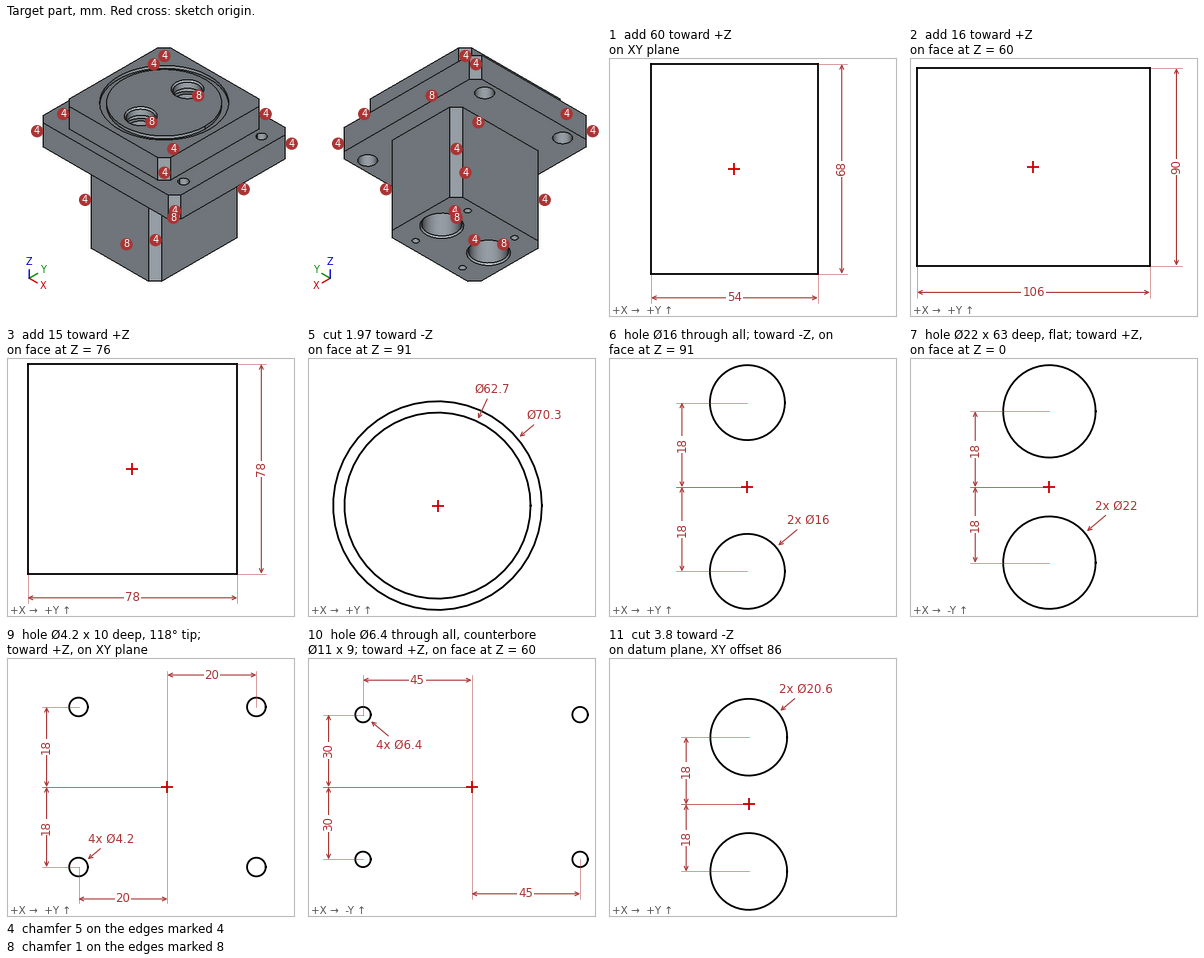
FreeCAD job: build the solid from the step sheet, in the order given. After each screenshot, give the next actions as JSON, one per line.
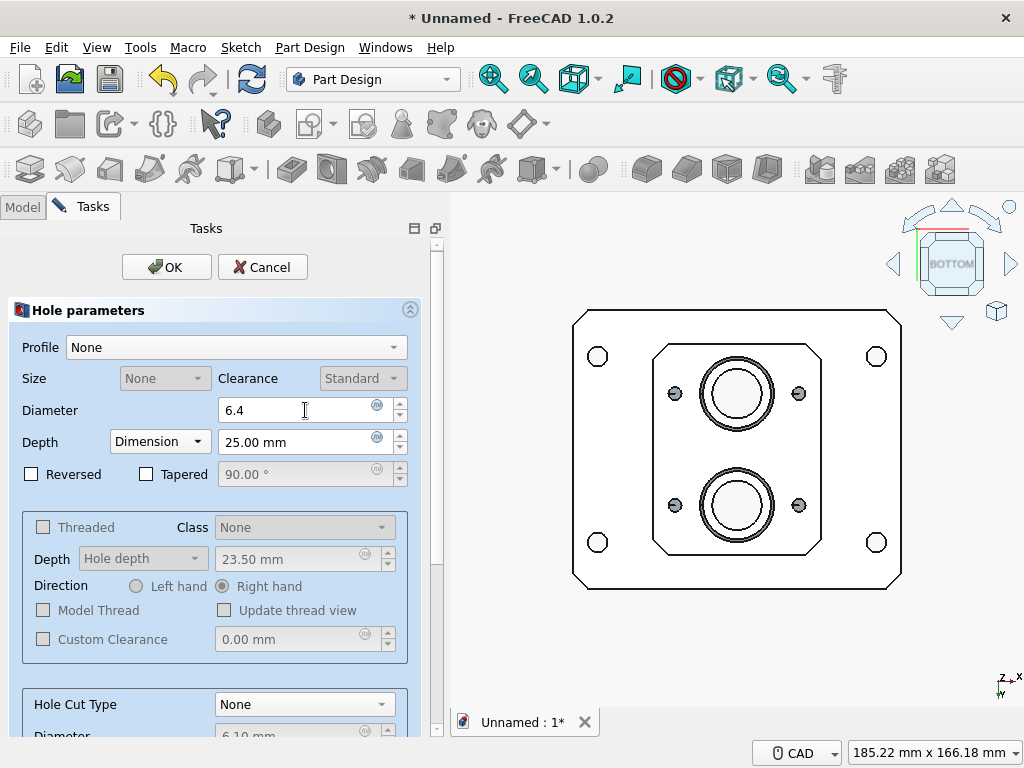
{"action": "left_click", "coordinate": [161, 442]}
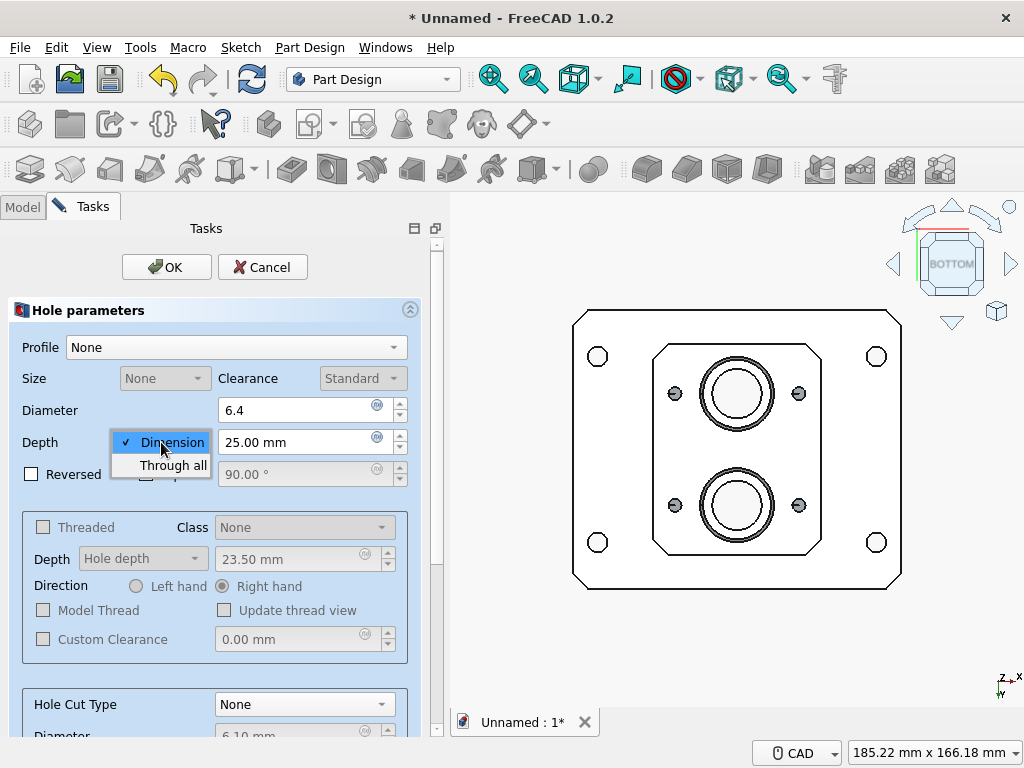
{"action": "left_click", "coordinate": [160, 466]}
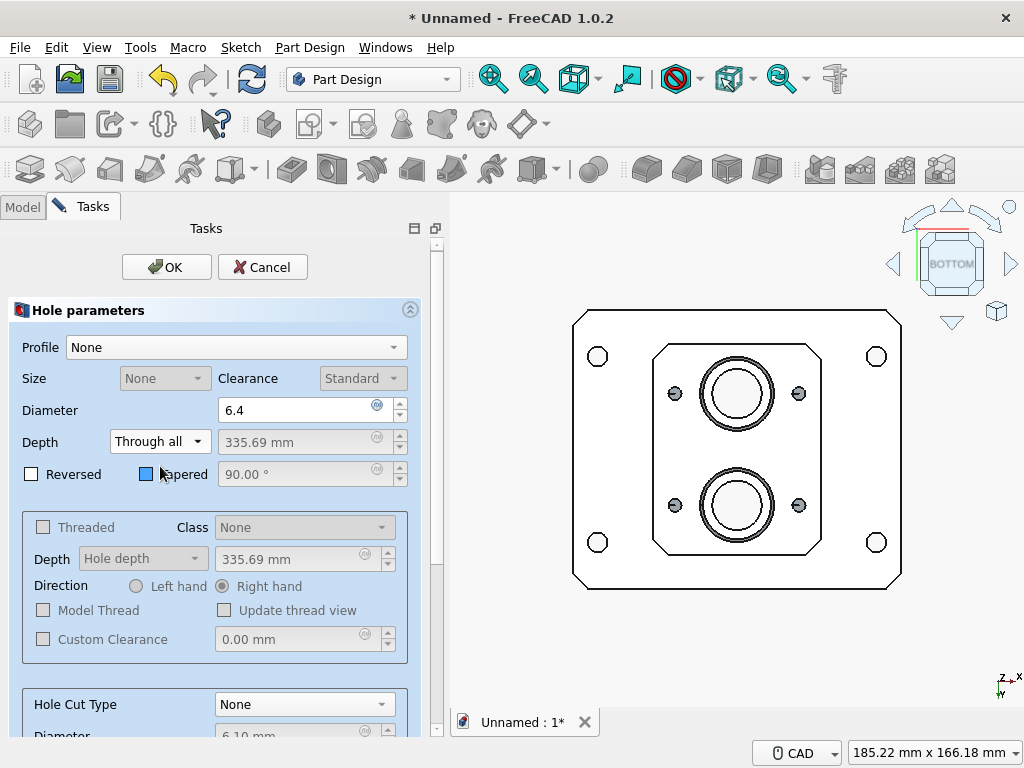
{"action": "left_click", "coordinate": [306, 704]}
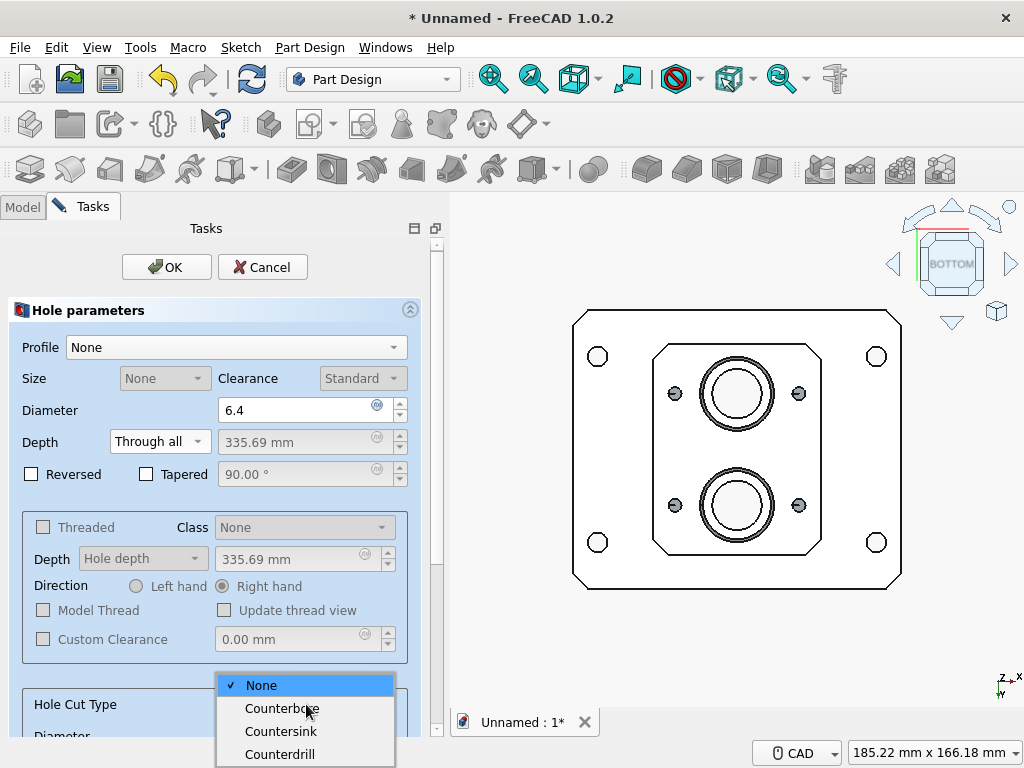
{"action": "left_click", "coordinate": [304, 708]}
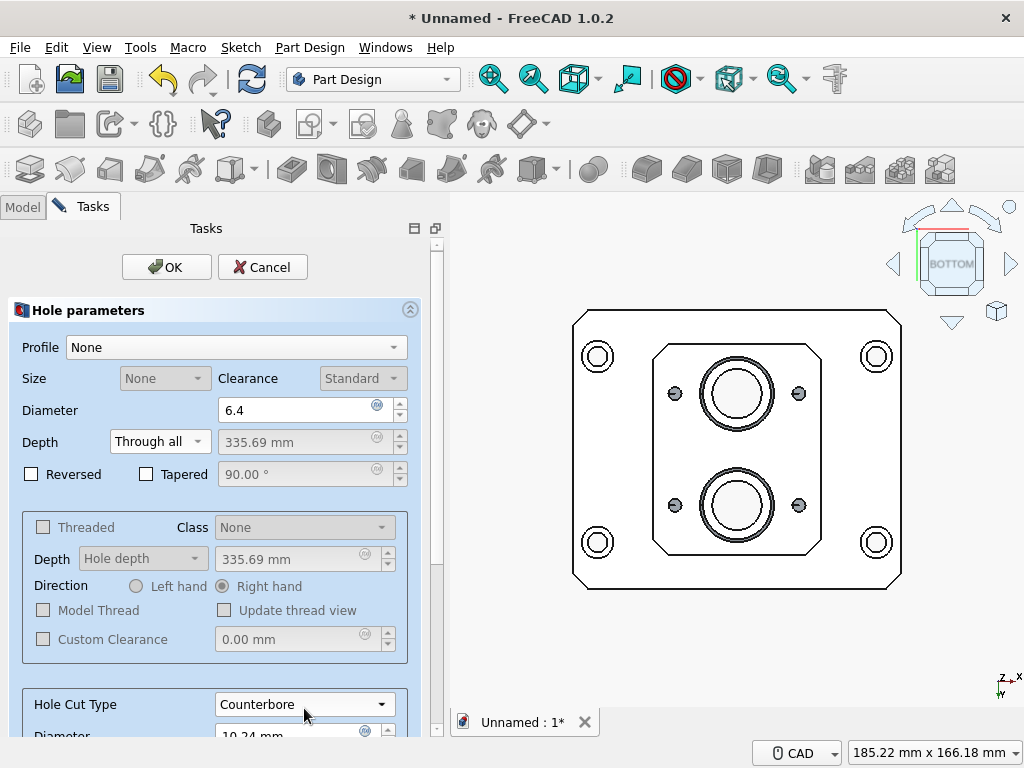
{"action": "scroll", "coordinate": [437, 487], "scroll_direction": "down", "scroll_amount": 2}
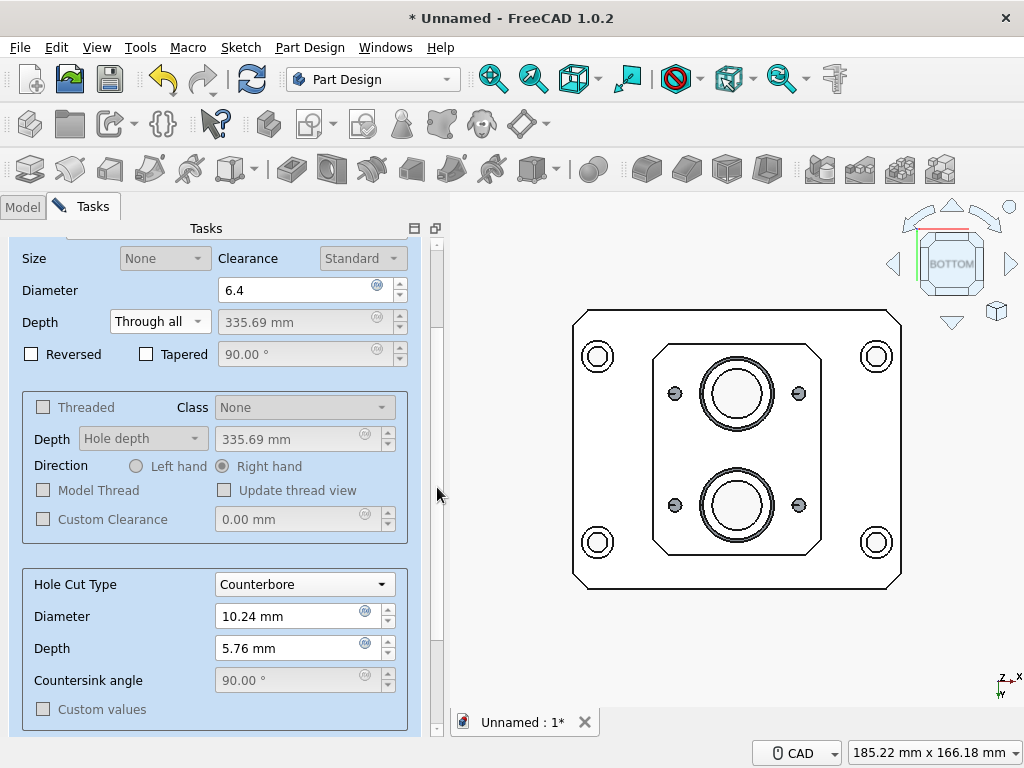
{"action": "triple_click", "coordinate": [298, 616]}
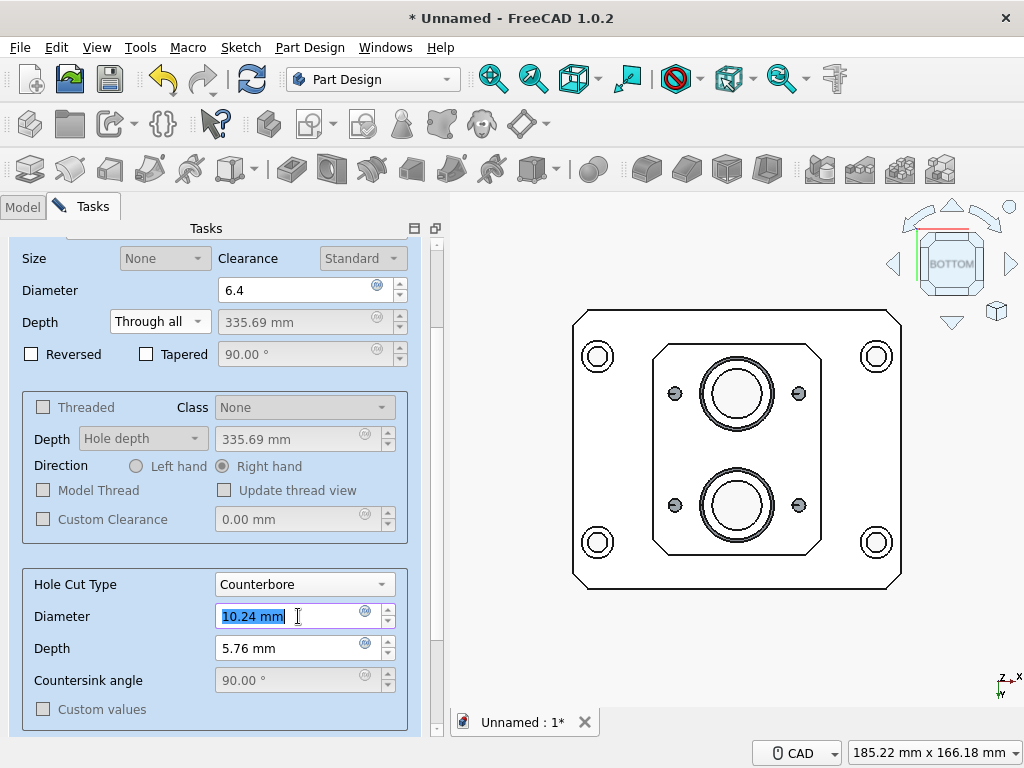
{"action": "type", "text": "11"}
{"action": "key", "text": "Tab"}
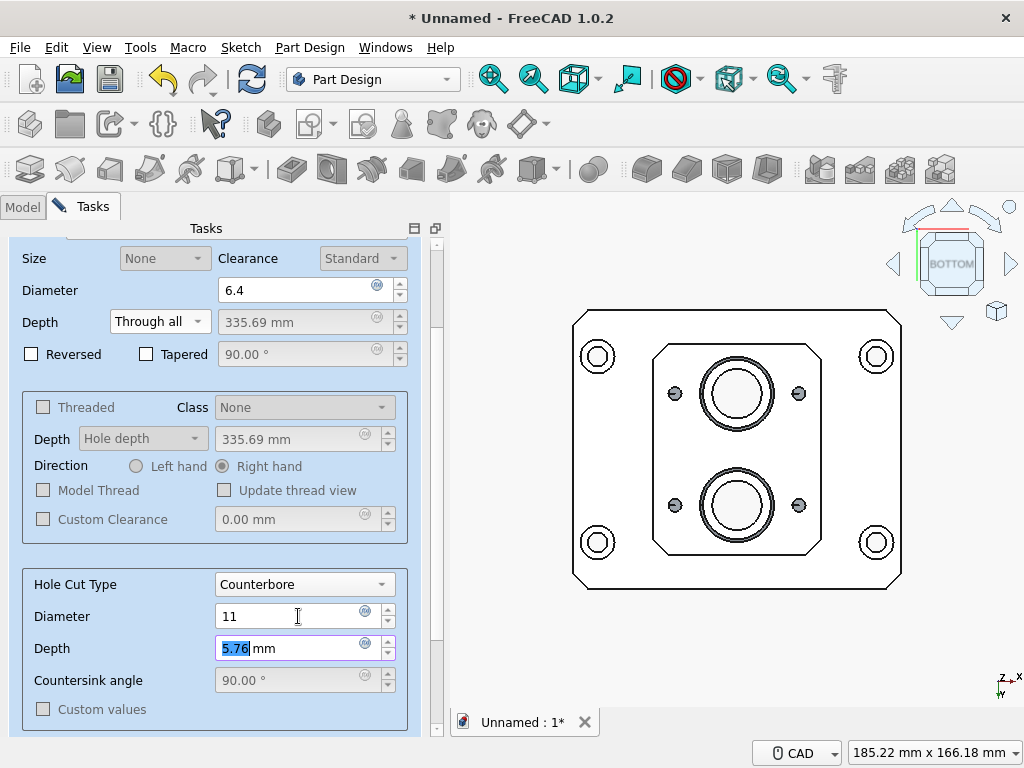
{"action": "type", "text": "9"}
{"action": "key", "text": "Tab"}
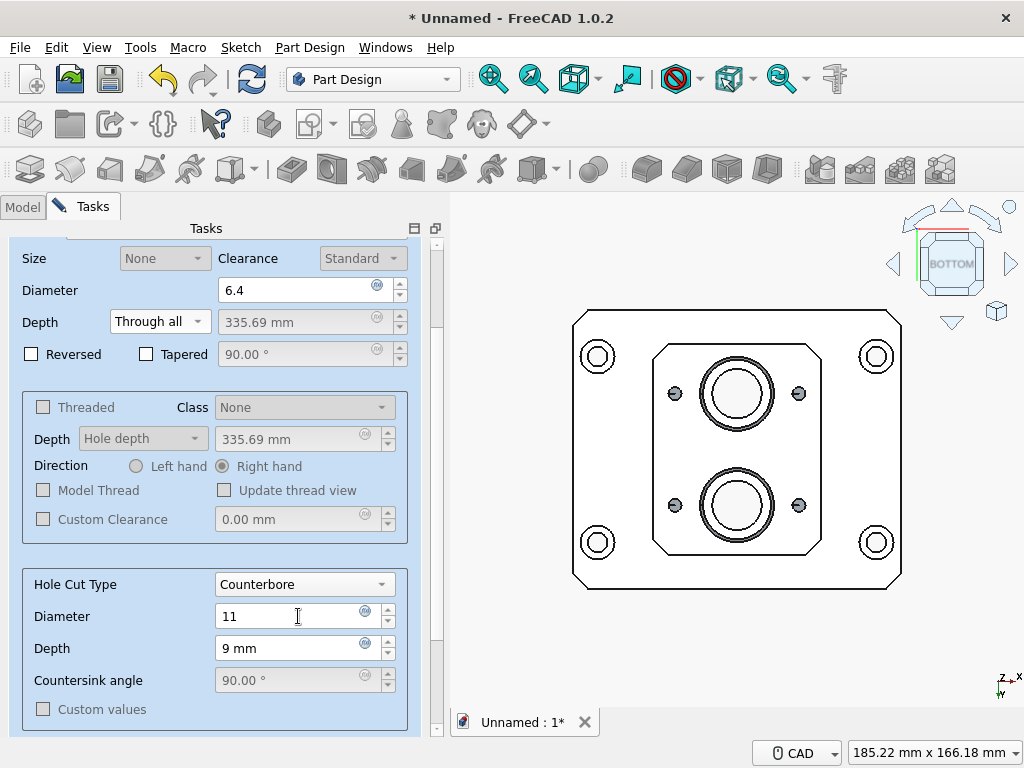
{"action": "scroll", "coordinate": [437, 487], "scroll_direction": "up", "scroll_amount": 3}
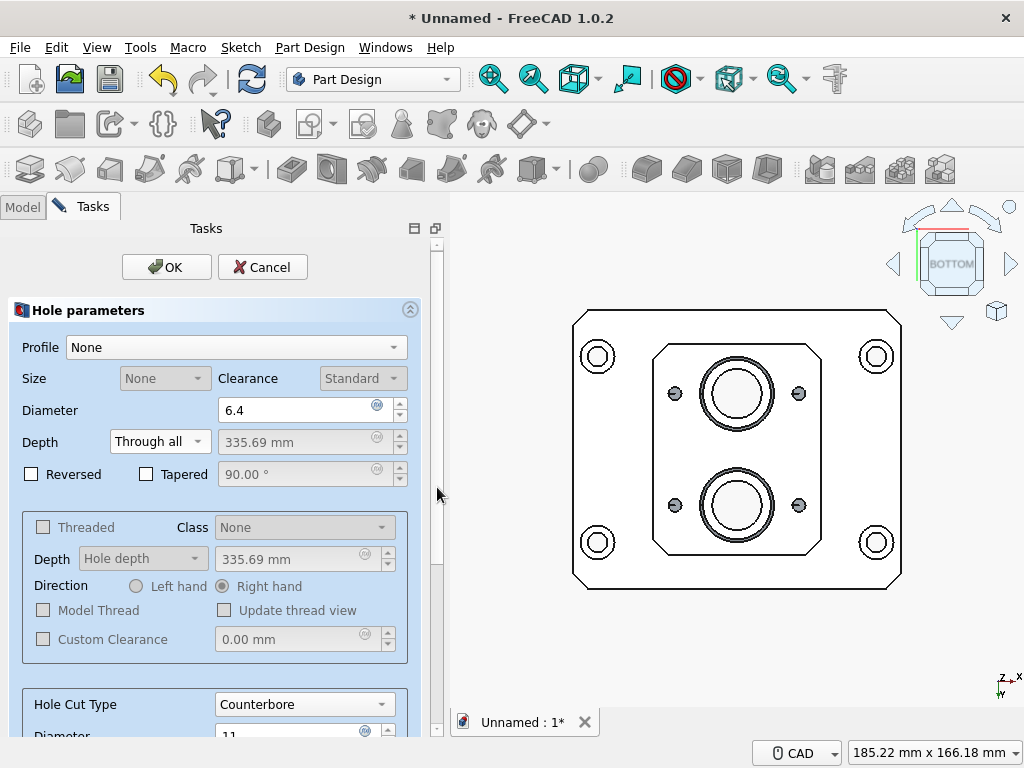
{"action": "left_click", "coordinate": [167, 267]}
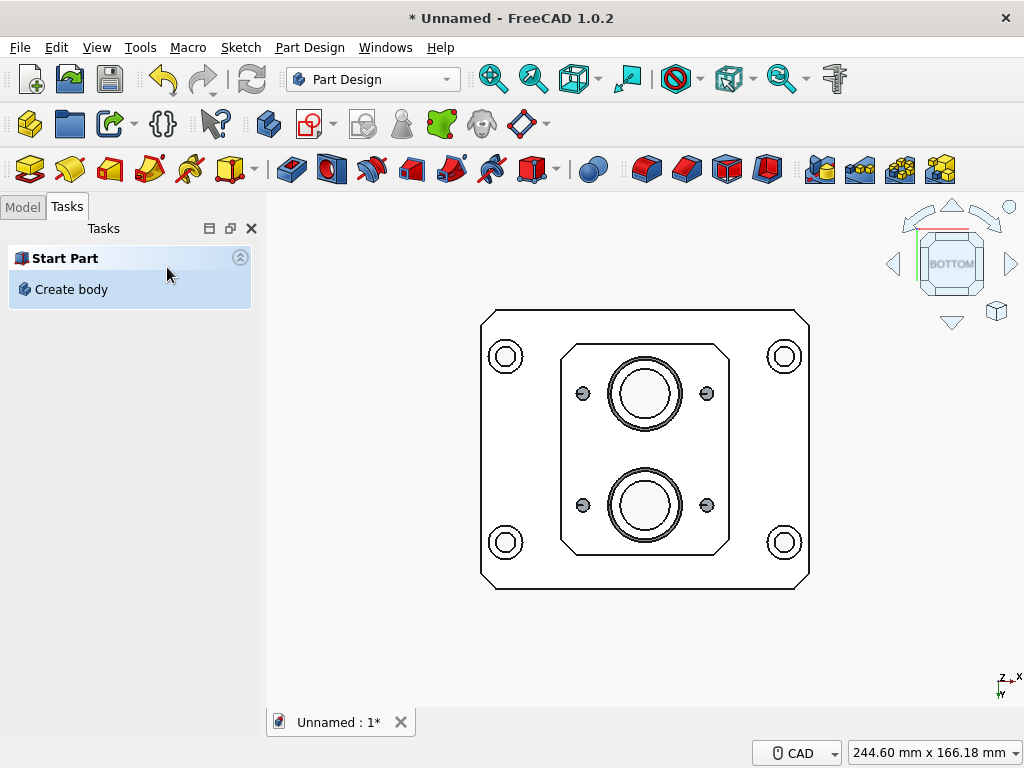
{"action": "left_click", "coordinate": [23, 206]}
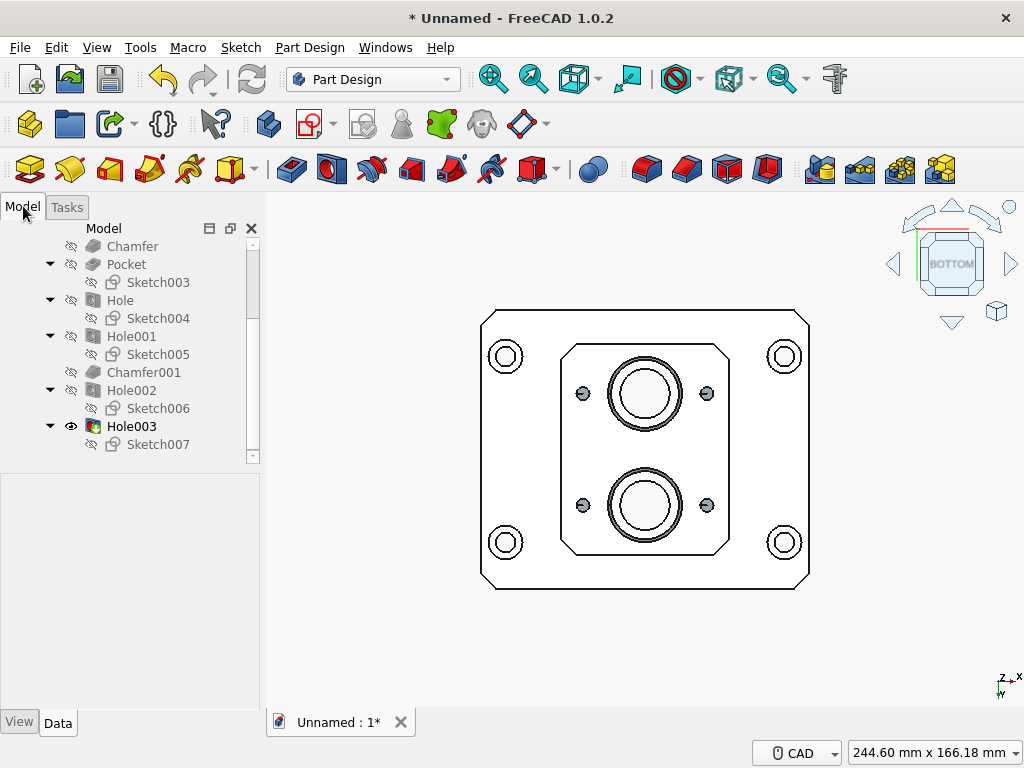
{"action": "scroll", "coordinate": [140, 350], "scroll_direction": "down", "scroll_amount": 3}